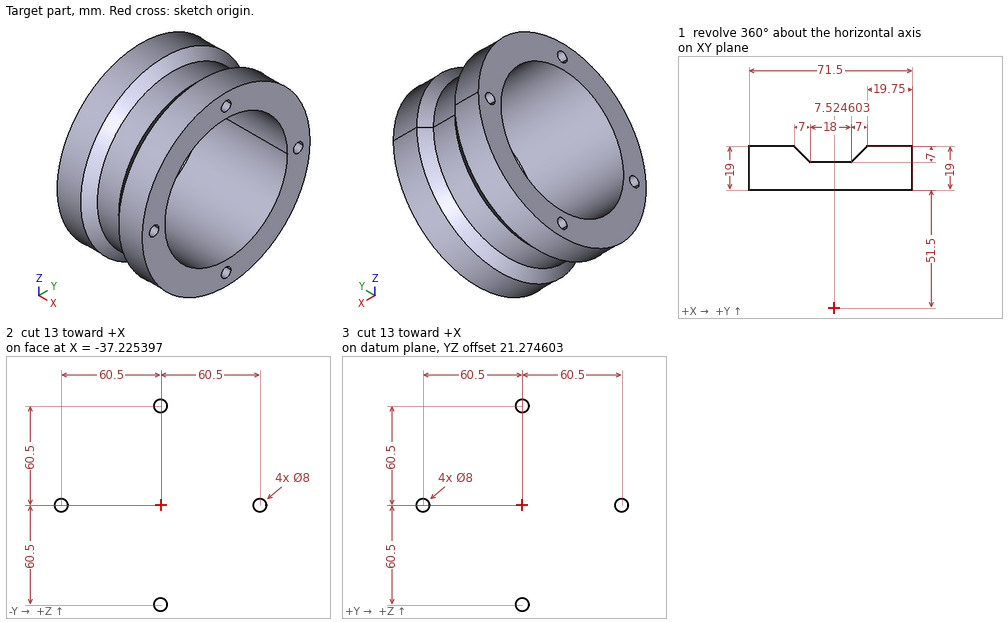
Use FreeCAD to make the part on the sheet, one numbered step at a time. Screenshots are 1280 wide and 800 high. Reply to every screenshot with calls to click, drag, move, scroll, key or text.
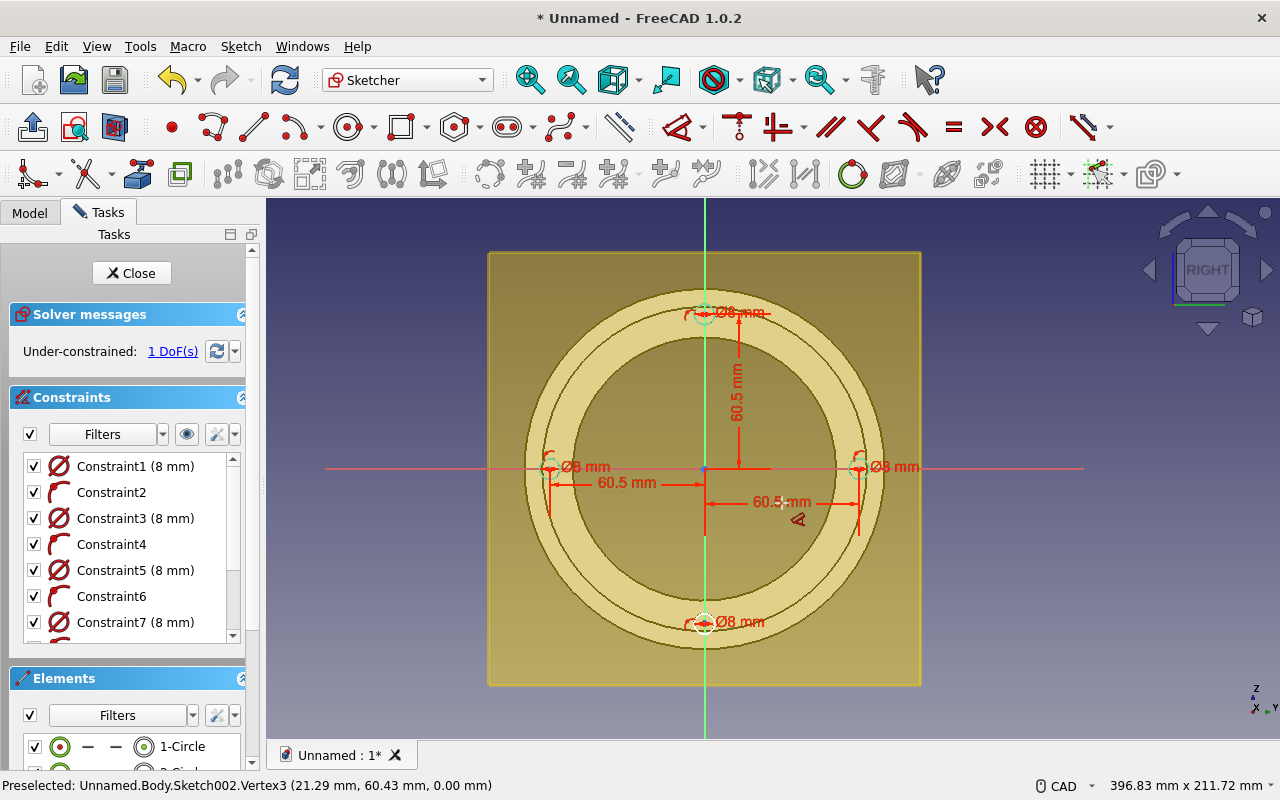
click(705, 624)
click(739, 547)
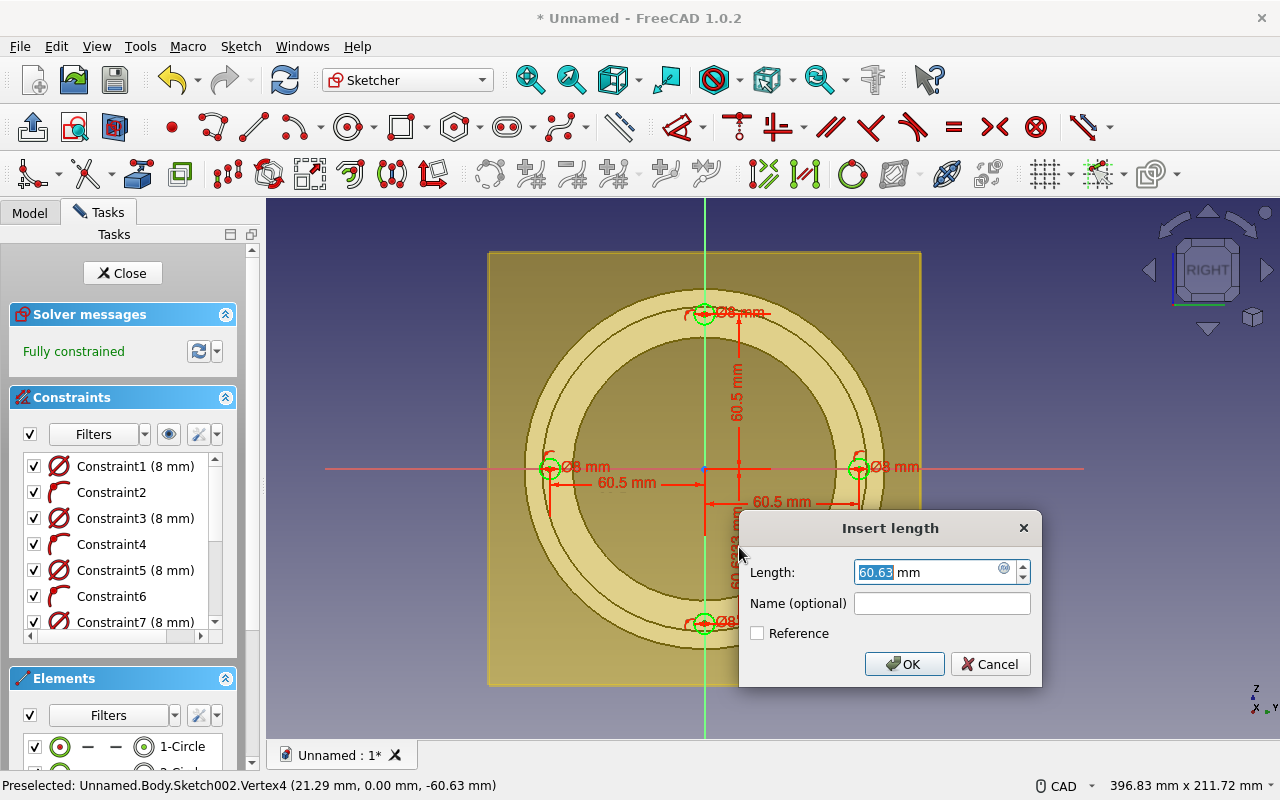
text(60.5)
key(Return)
key(Escape)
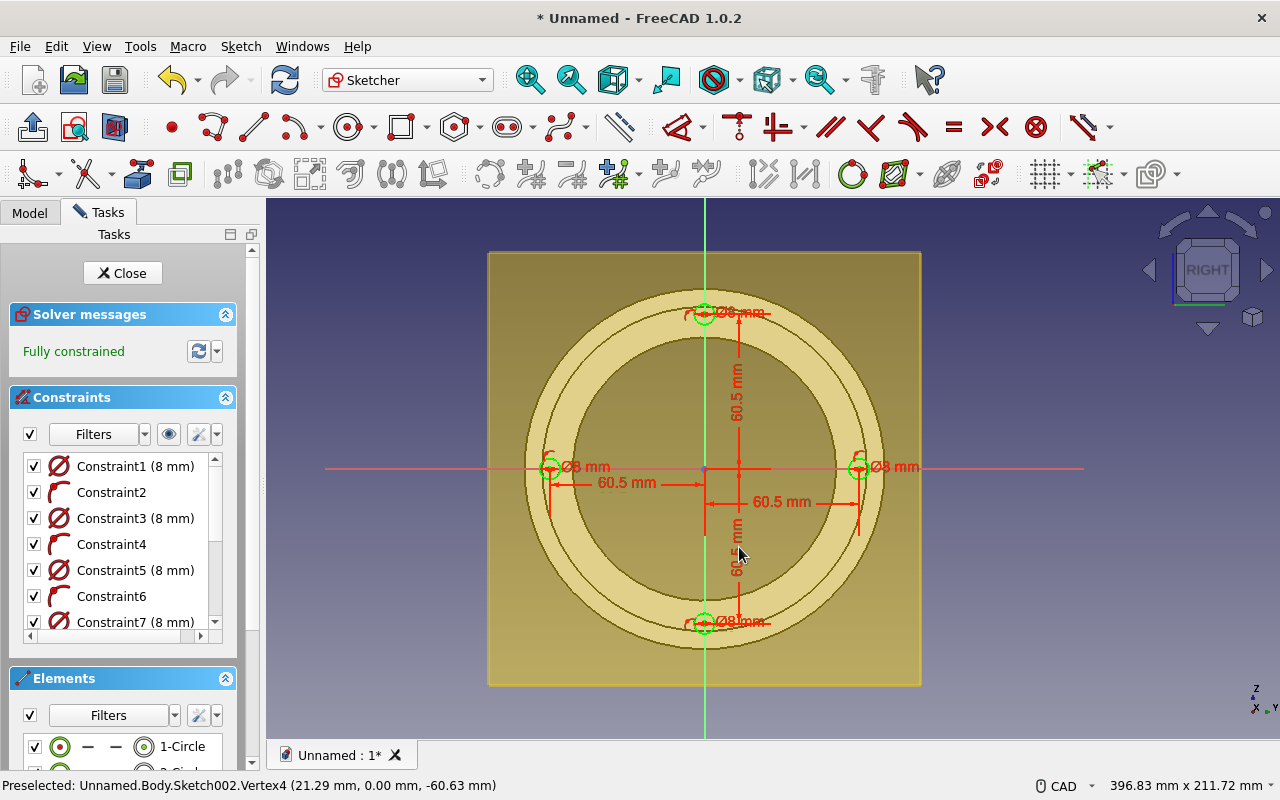
click(123, 273)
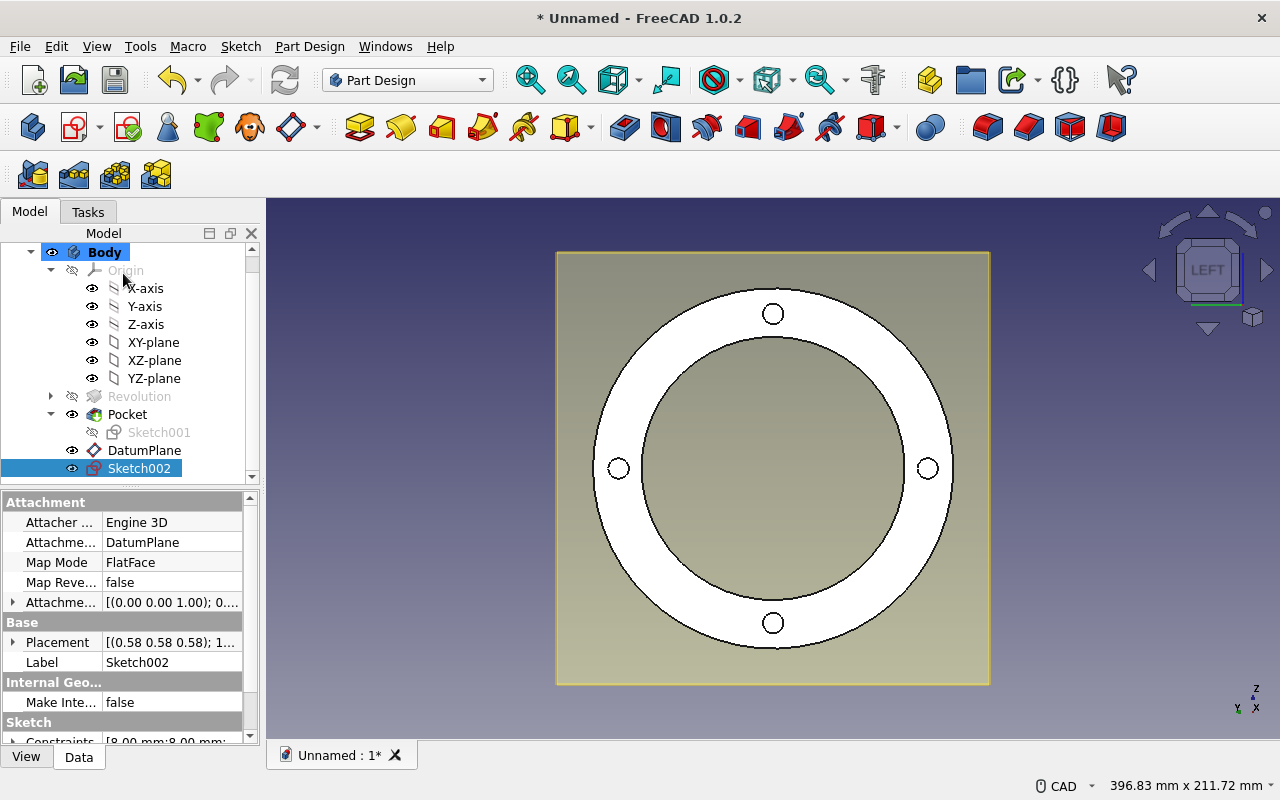
click(625, 128)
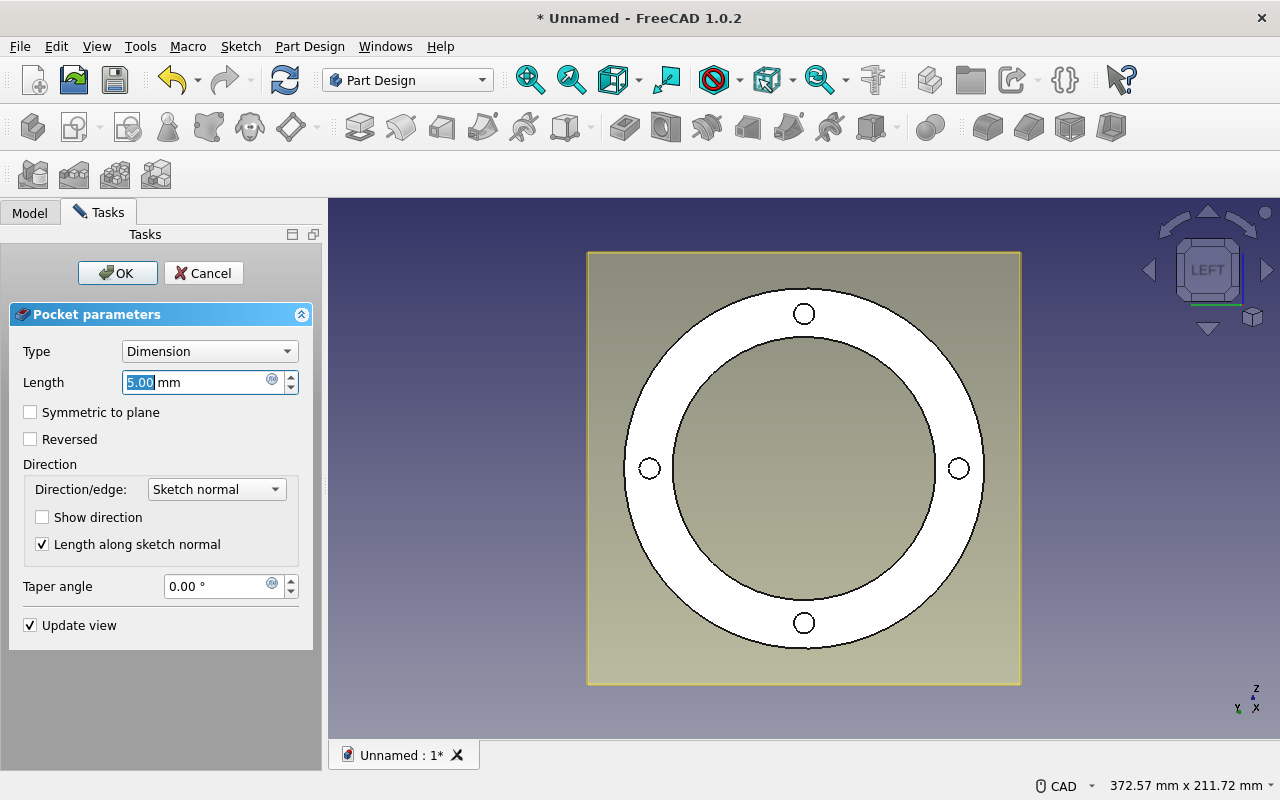
text(13)
key(Tab)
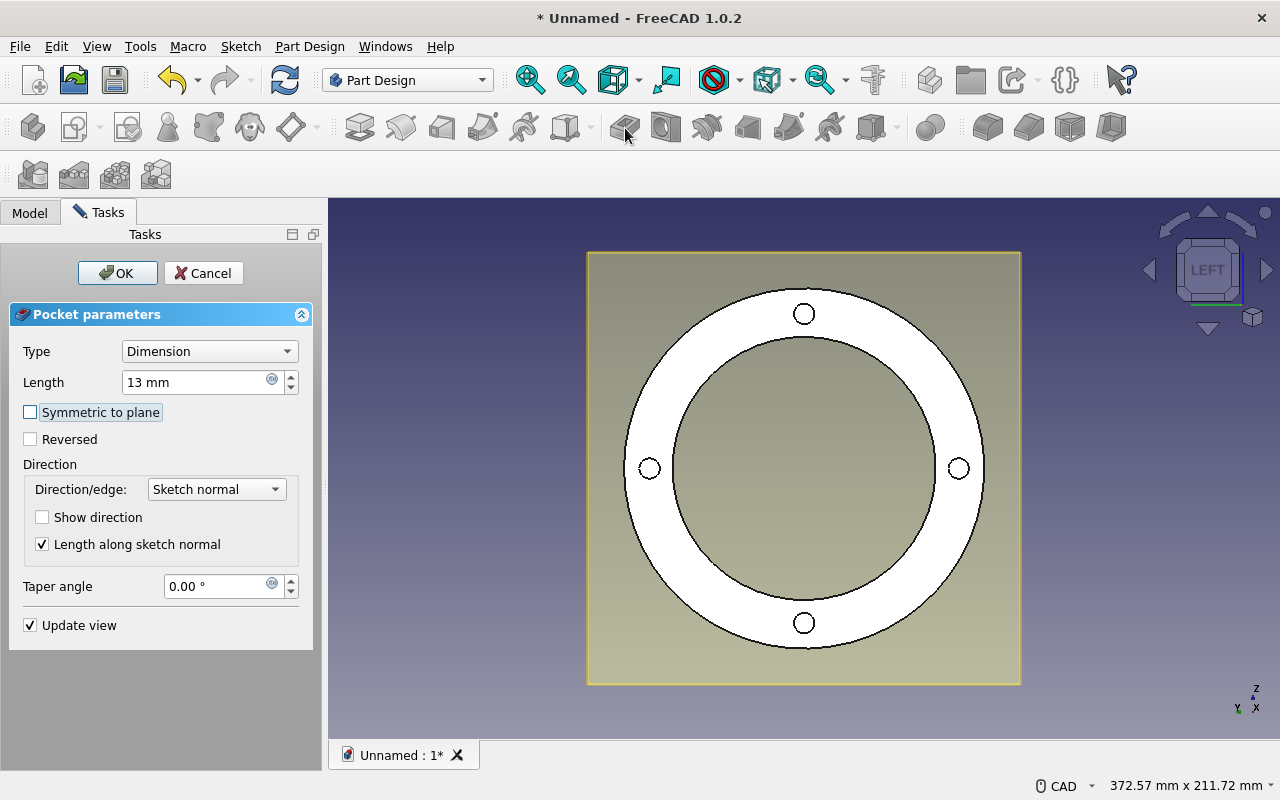
click(31, 439)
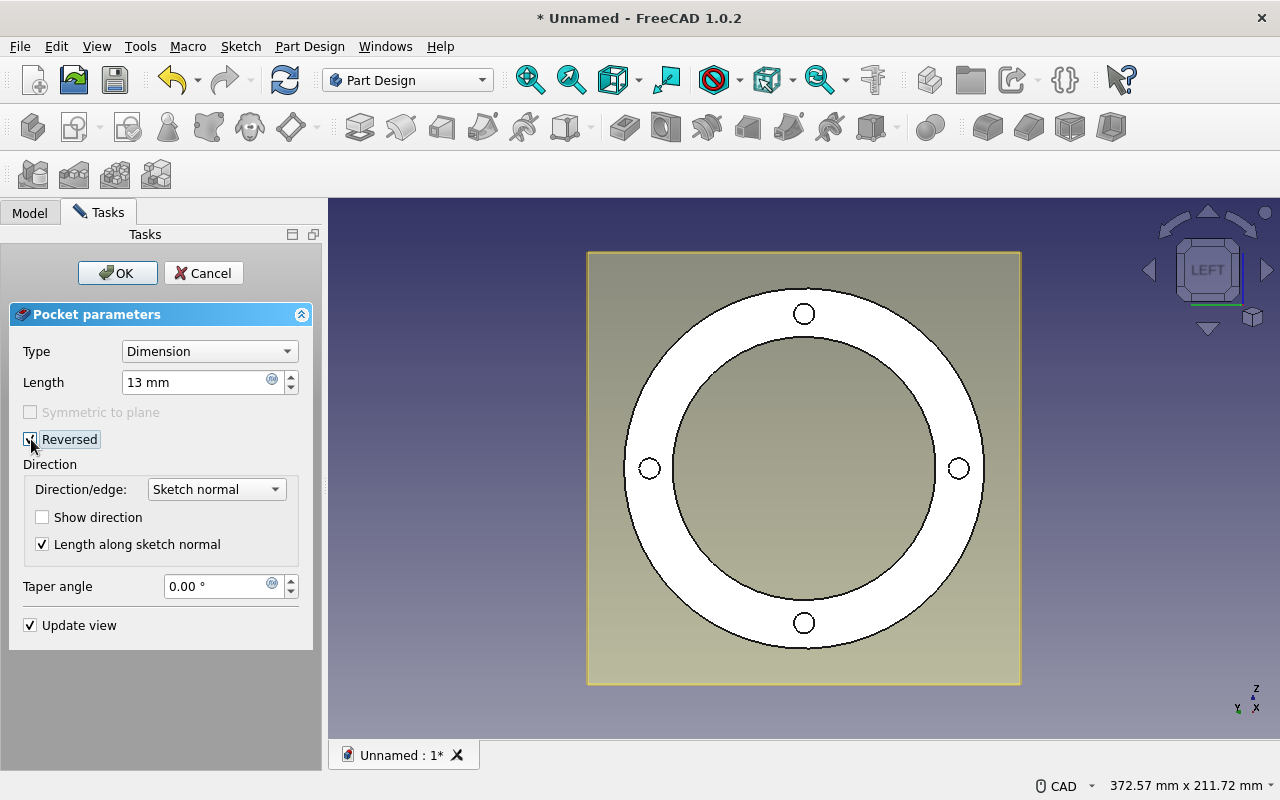
click(118, 273)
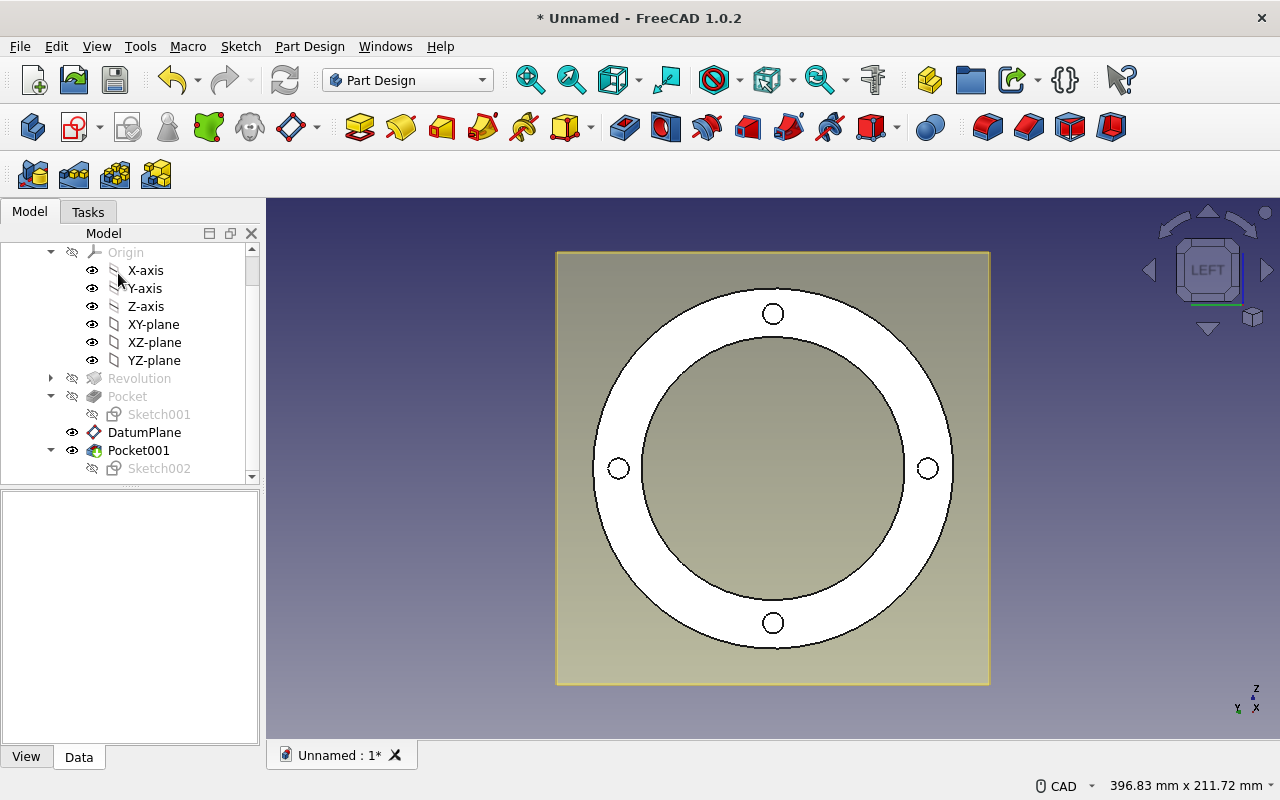
click(117, 432)
key(space)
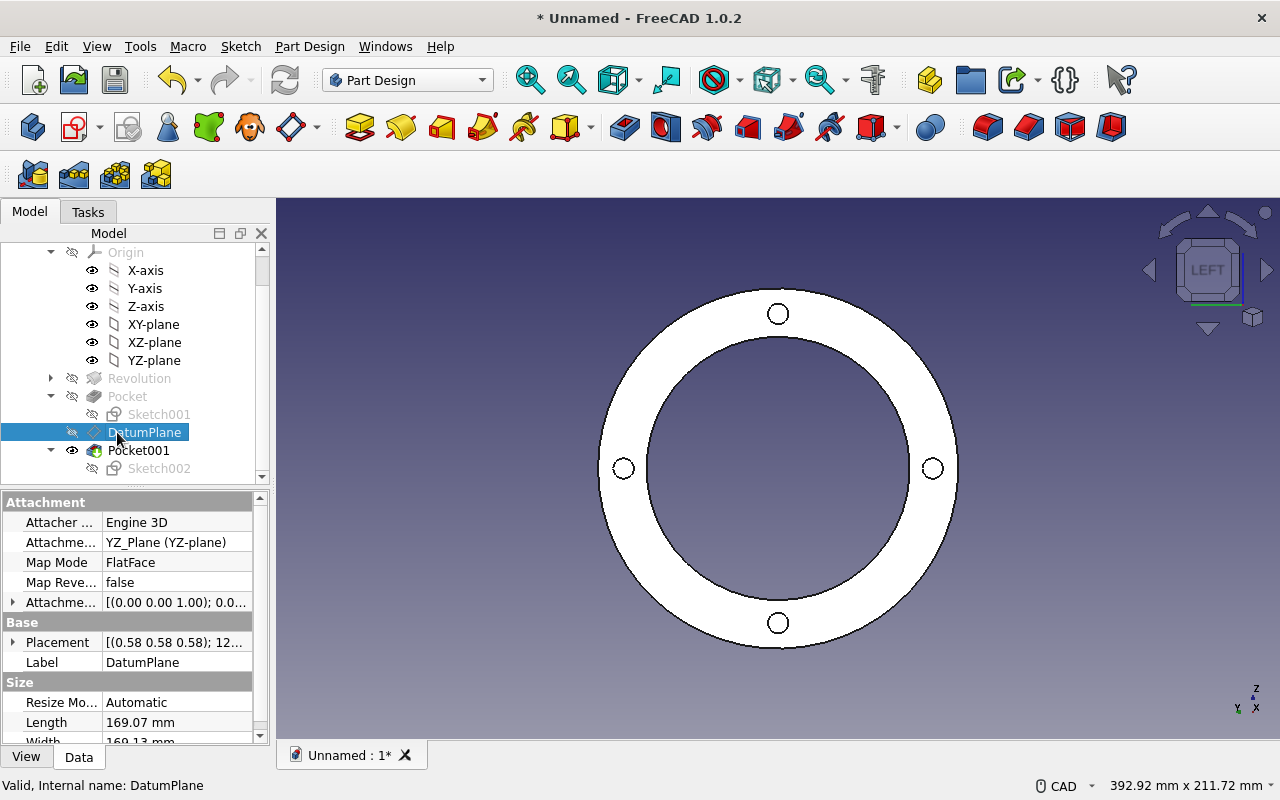
key(0)